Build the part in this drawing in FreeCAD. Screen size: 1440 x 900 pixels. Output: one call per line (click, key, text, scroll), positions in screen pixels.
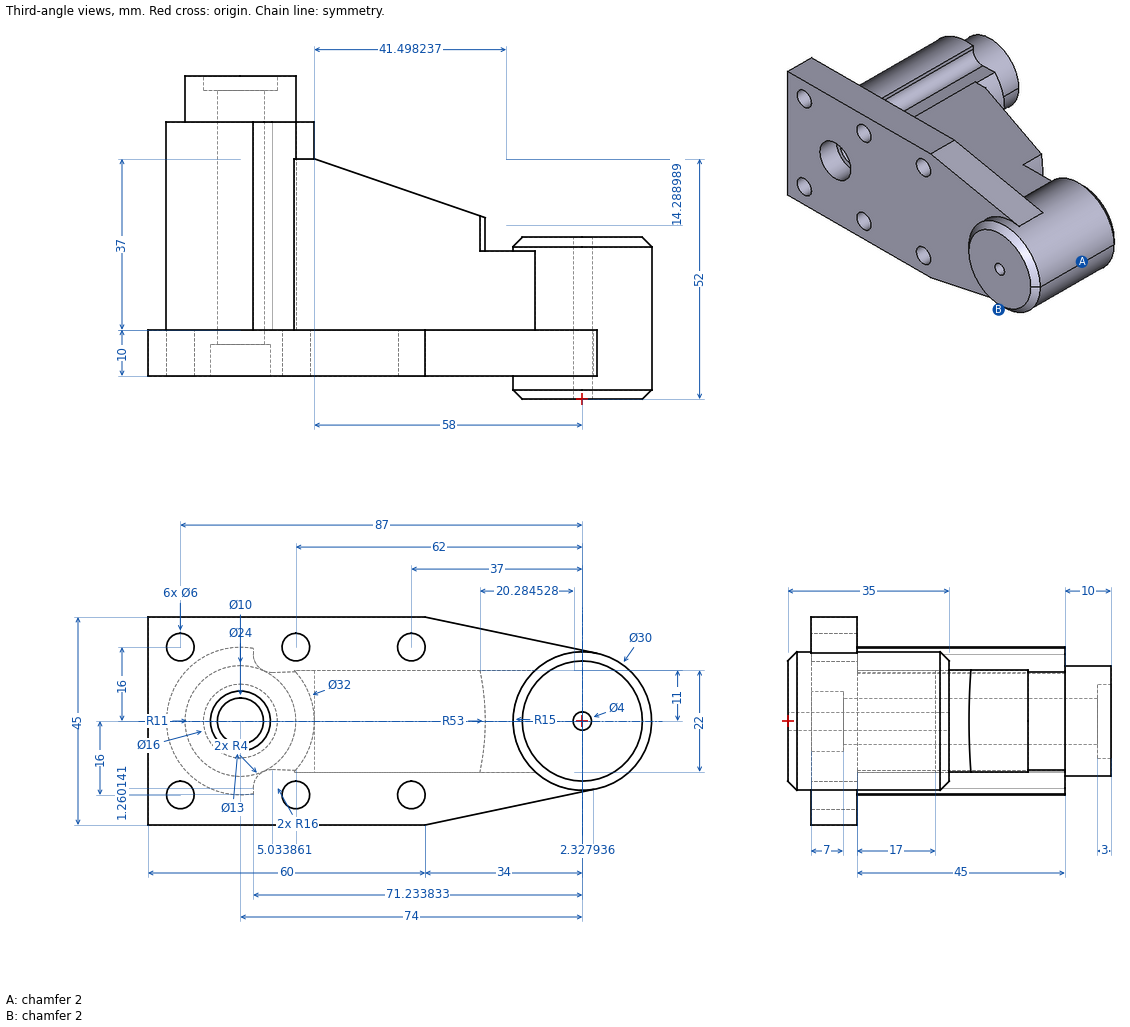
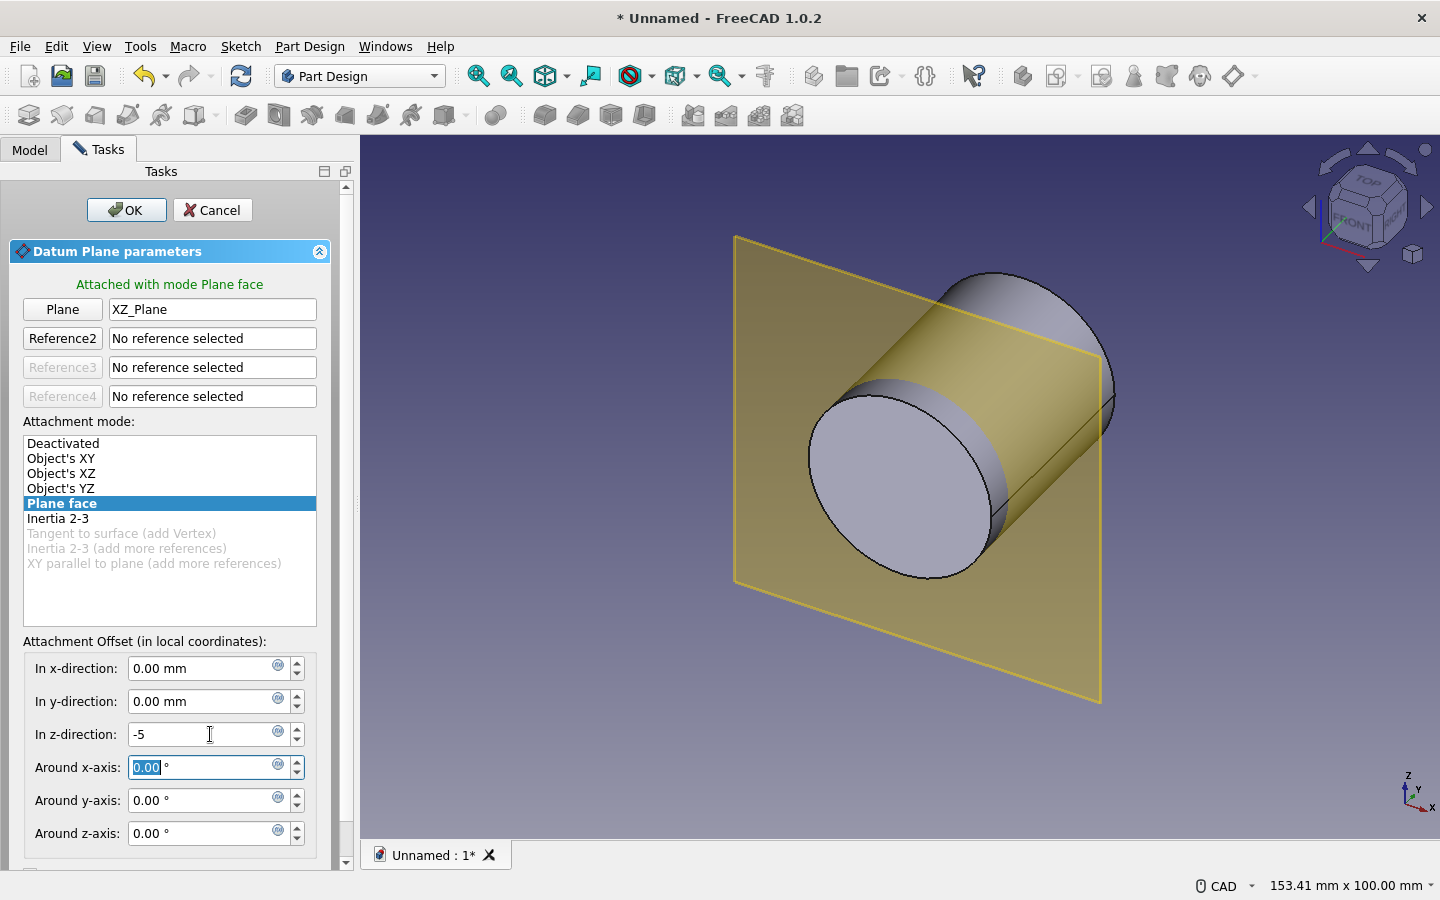
click(127, 210)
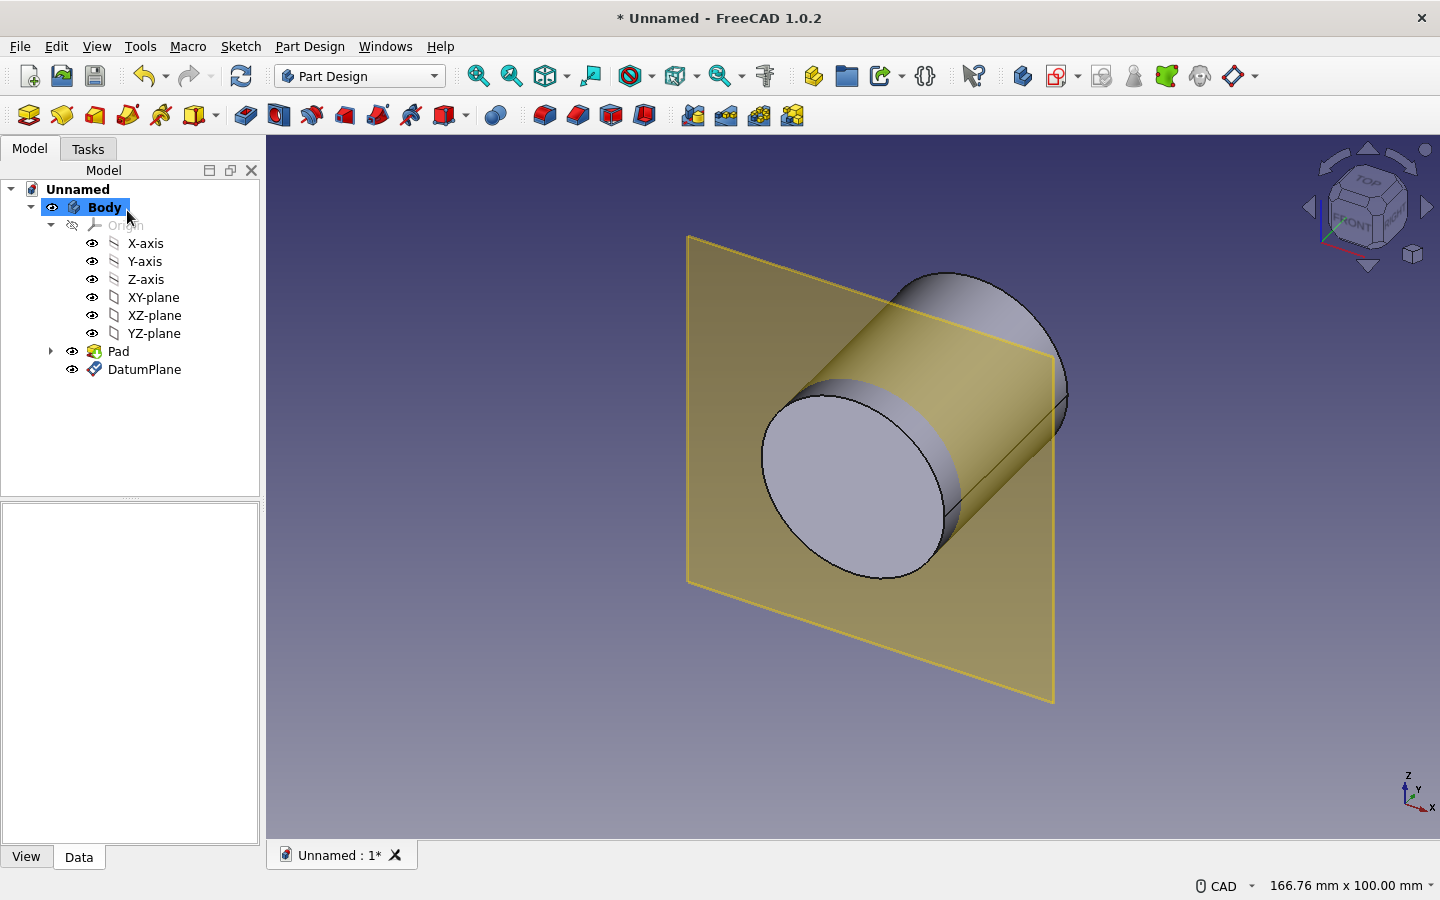
click(117, 369)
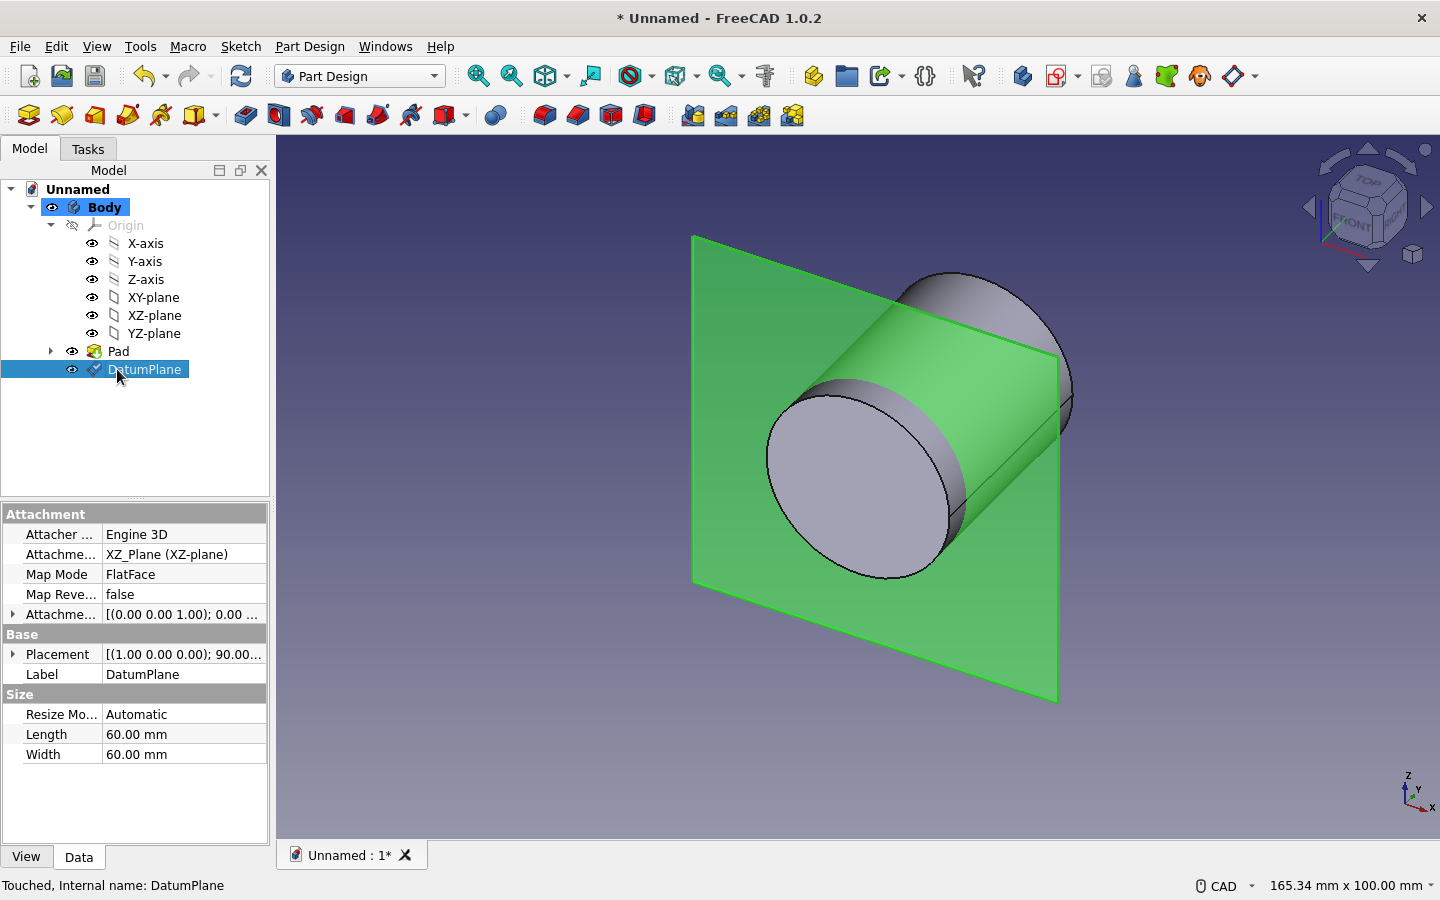
click(1056, 76)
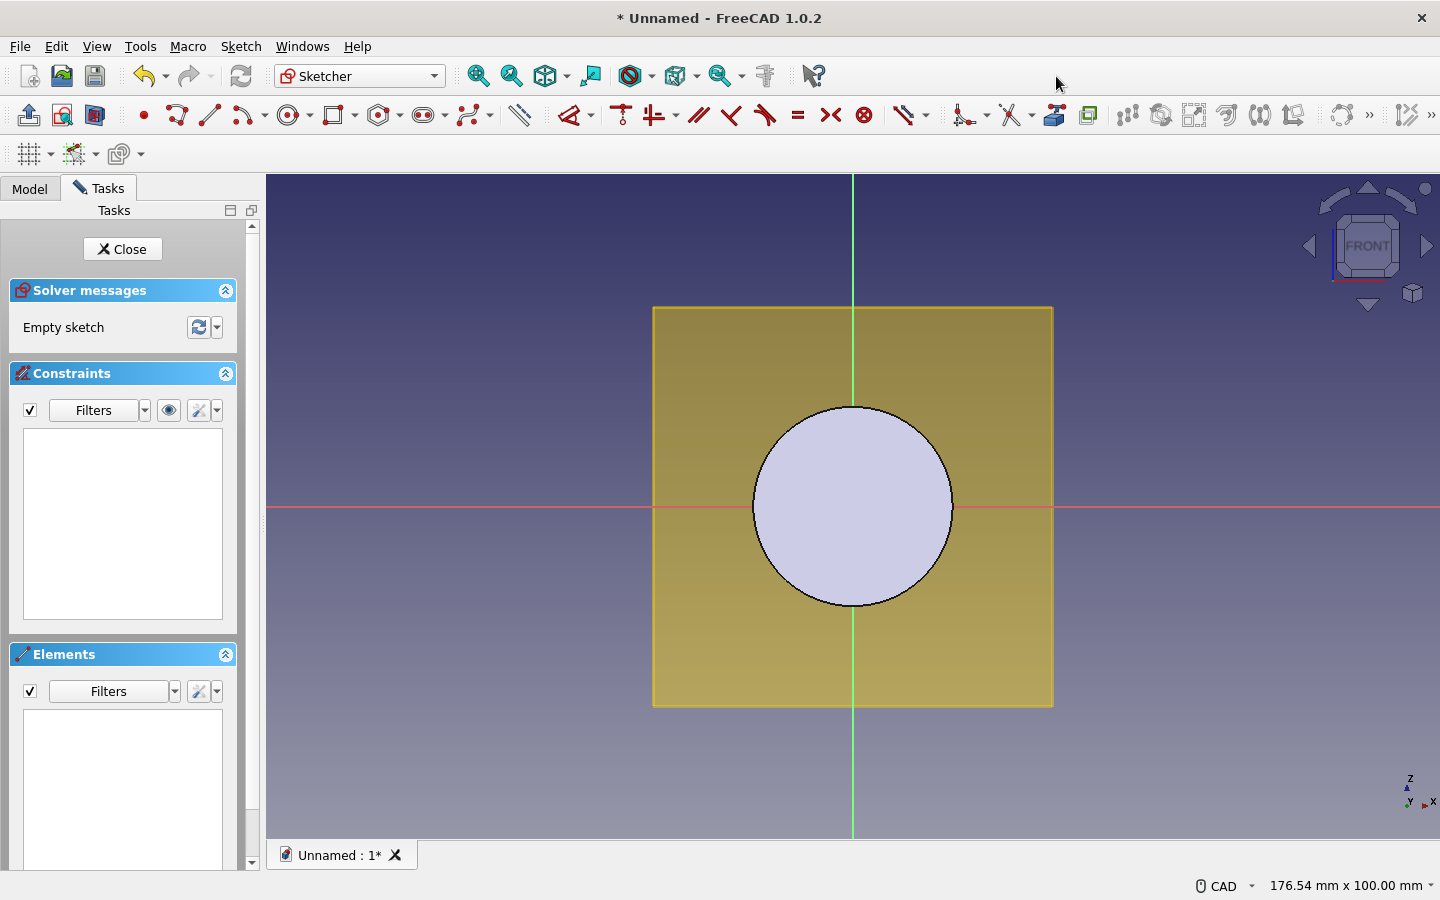
click(95, 116)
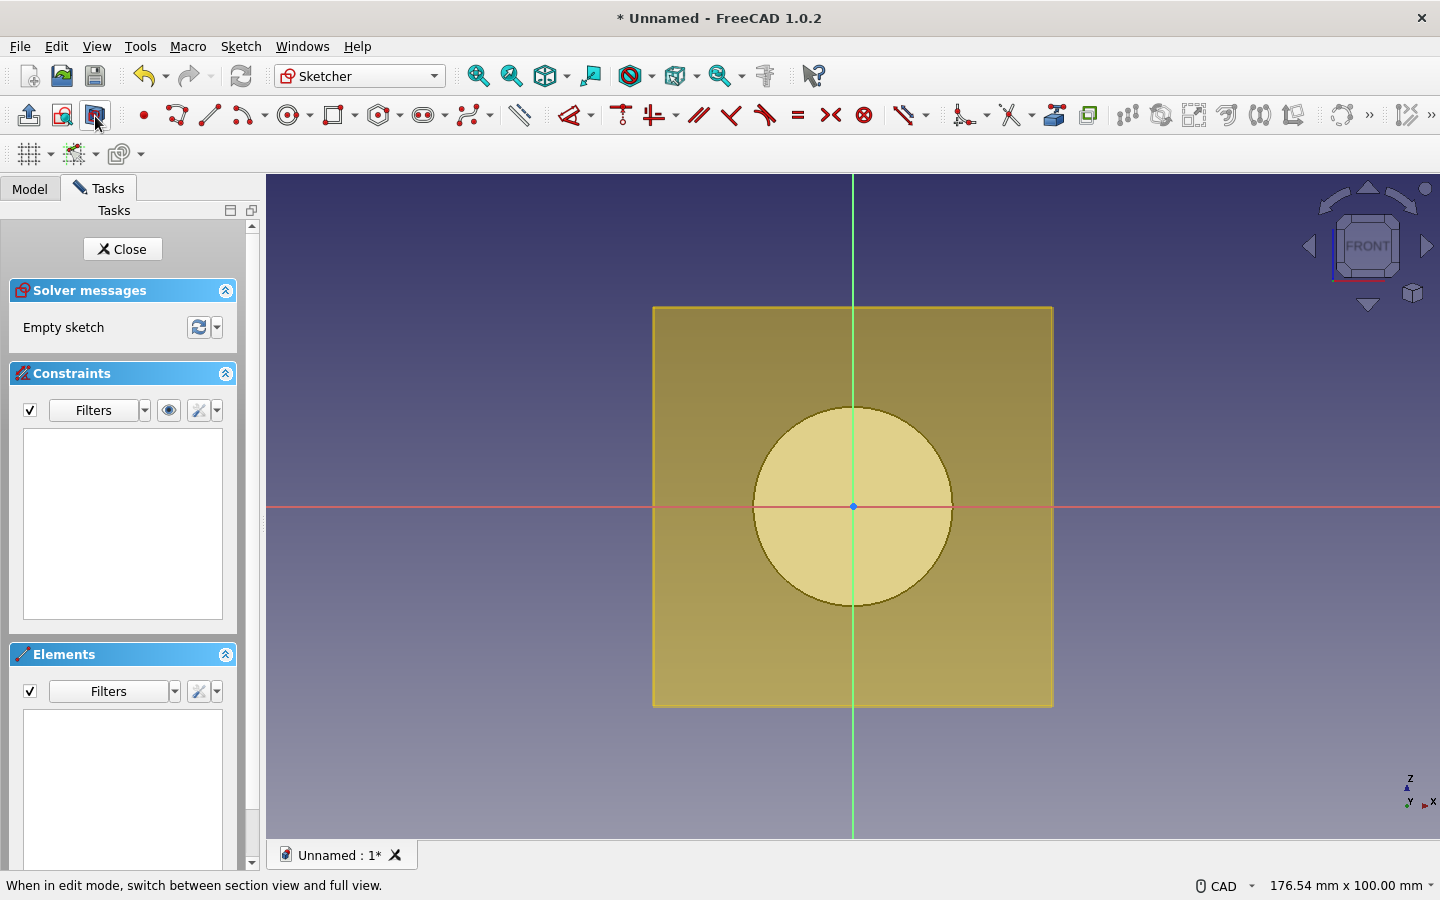
scroll(1275, 507, down, 1)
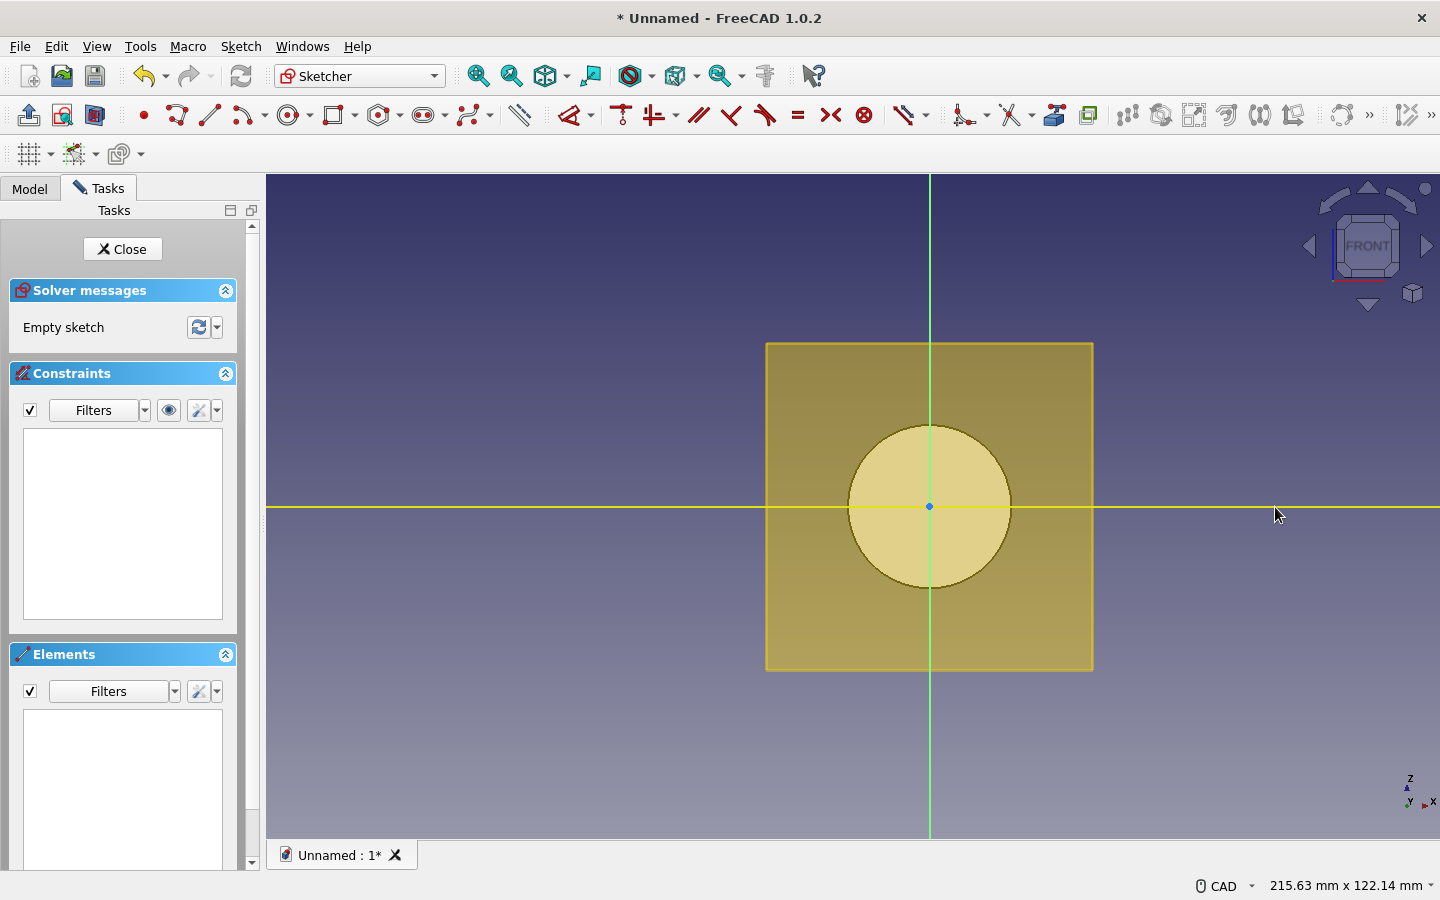
click(177, 116)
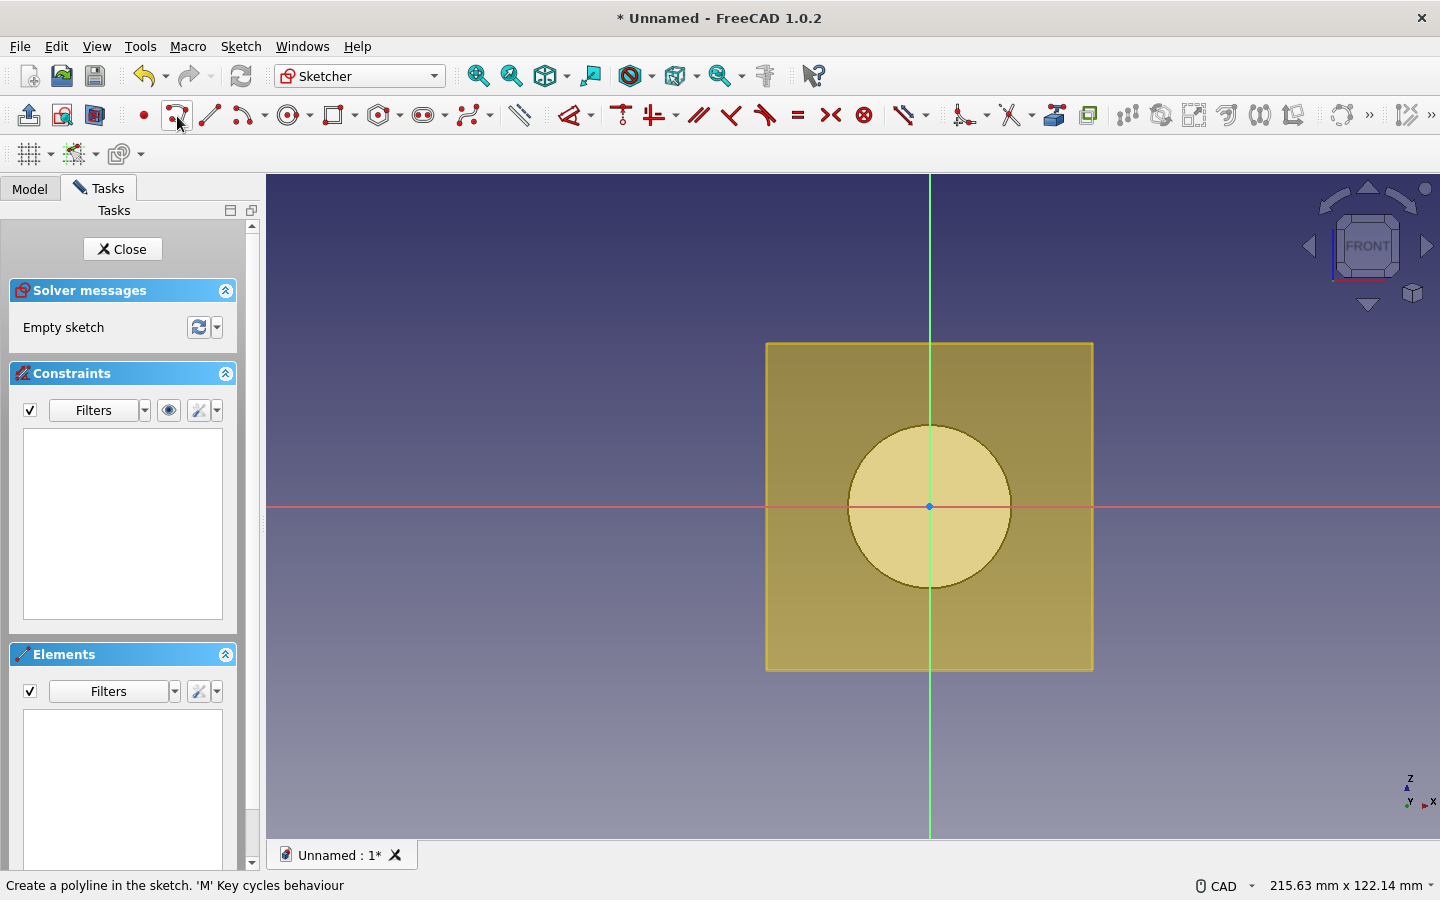
scroll(942, 587, up, 2)